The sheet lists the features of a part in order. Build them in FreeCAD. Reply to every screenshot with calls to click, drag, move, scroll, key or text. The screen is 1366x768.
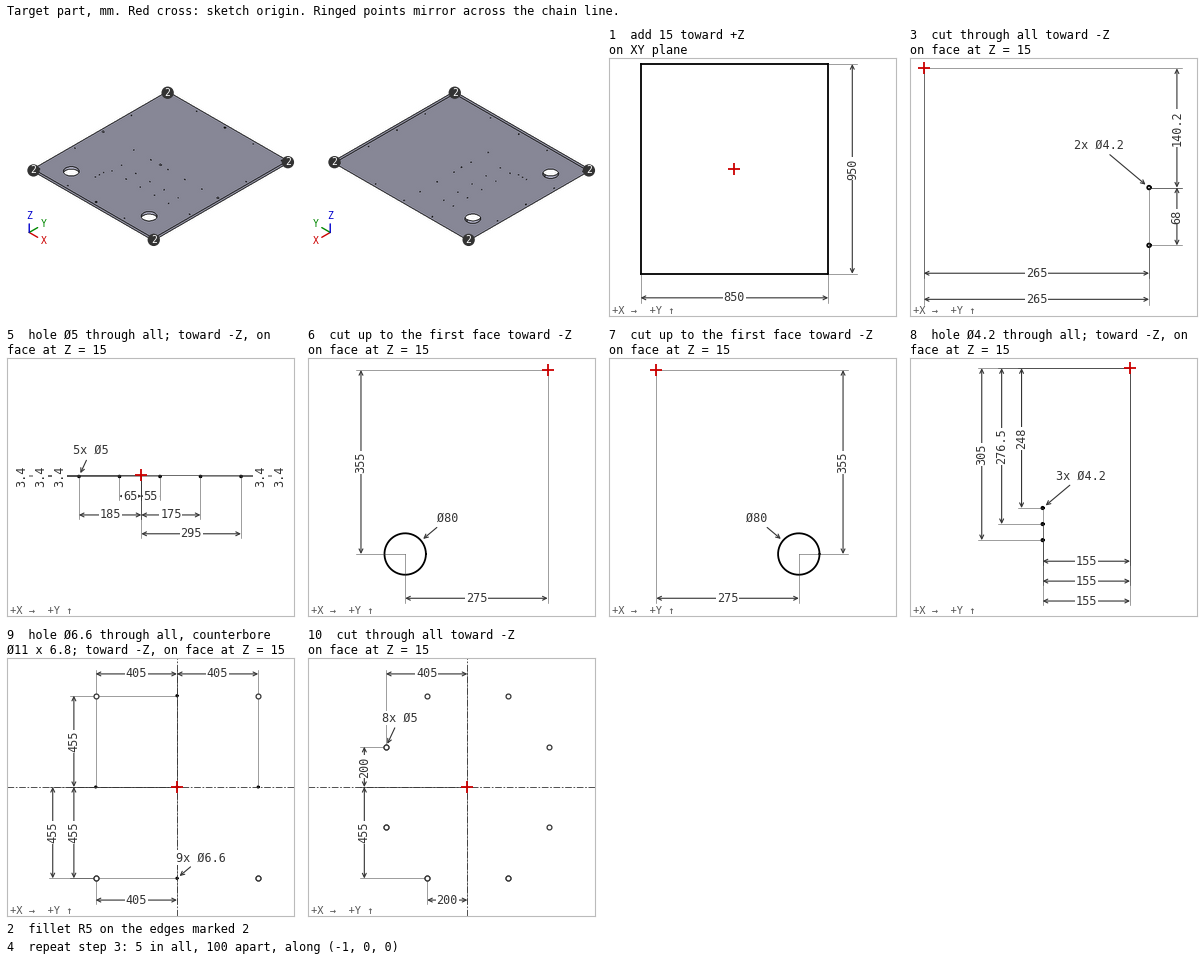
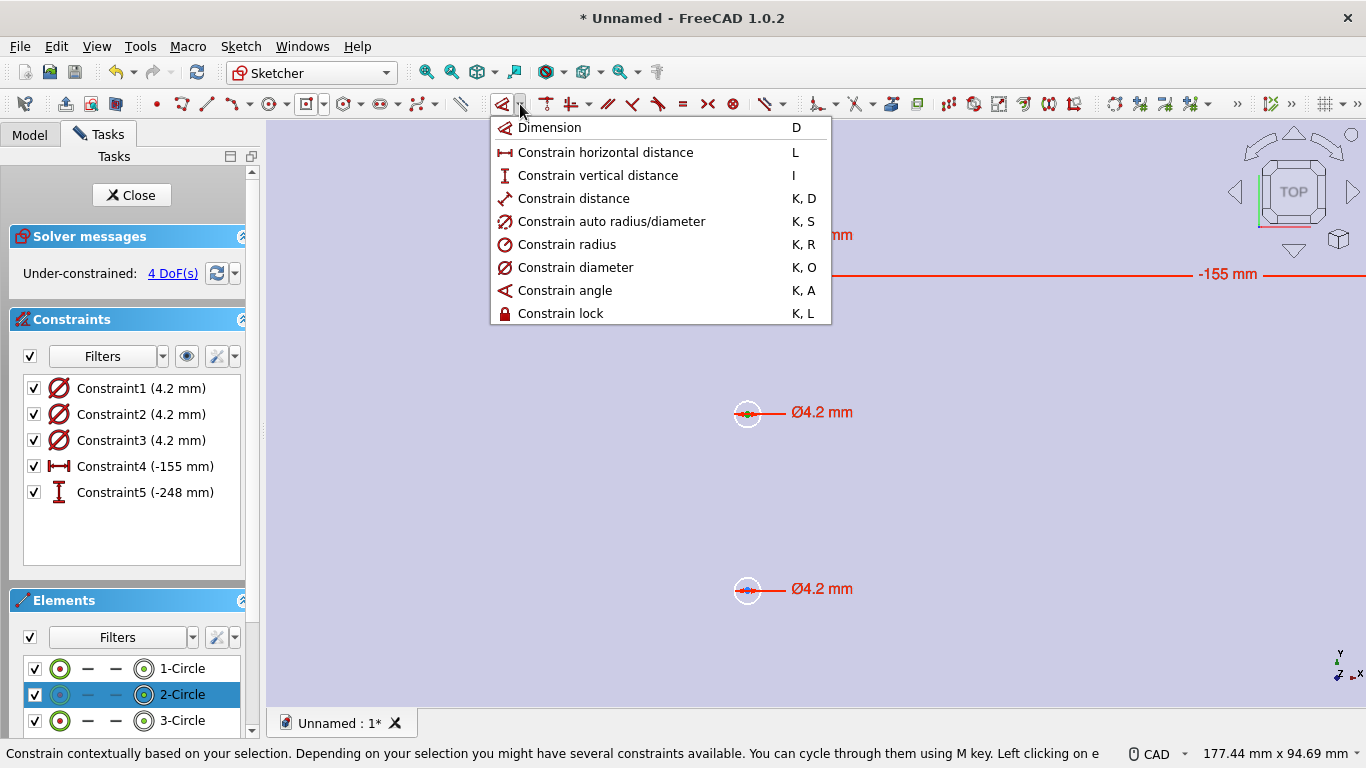
click(661, 152)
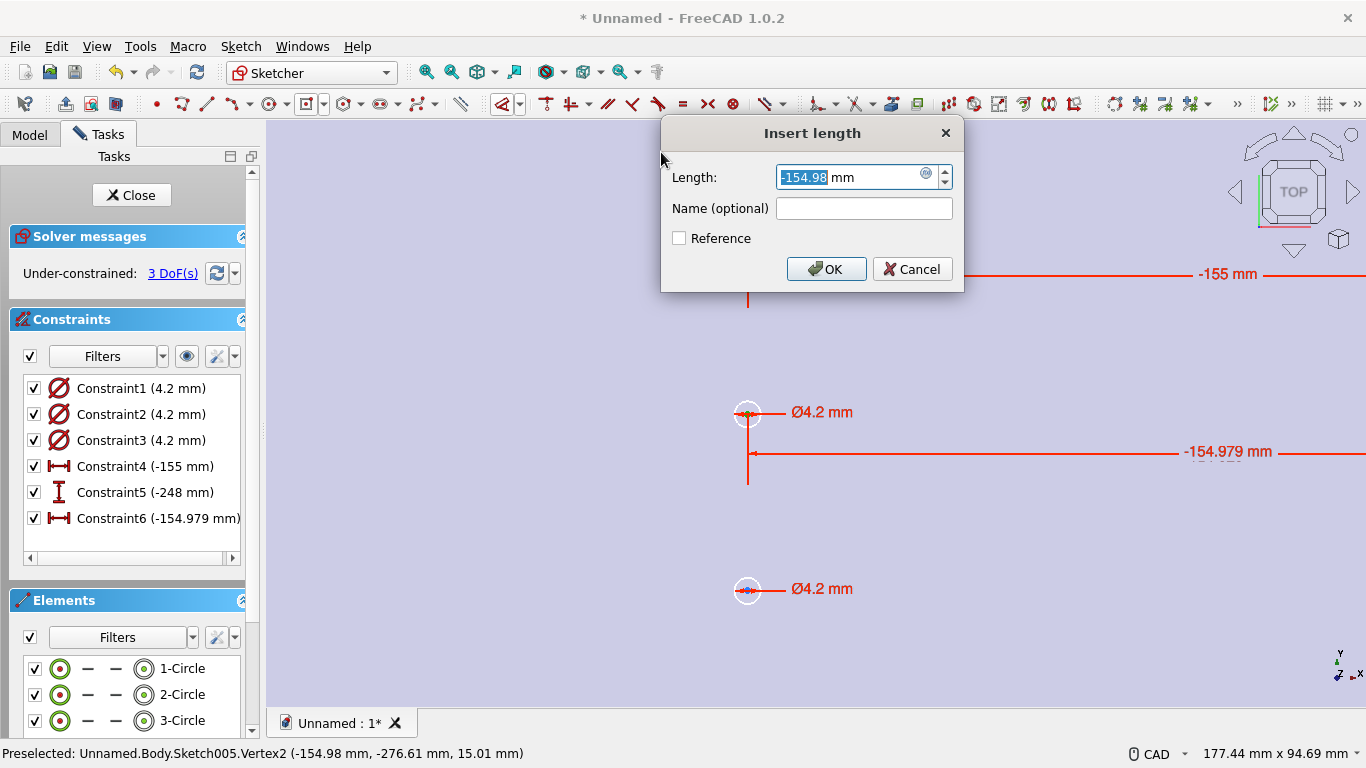
text(-155)
key(Return)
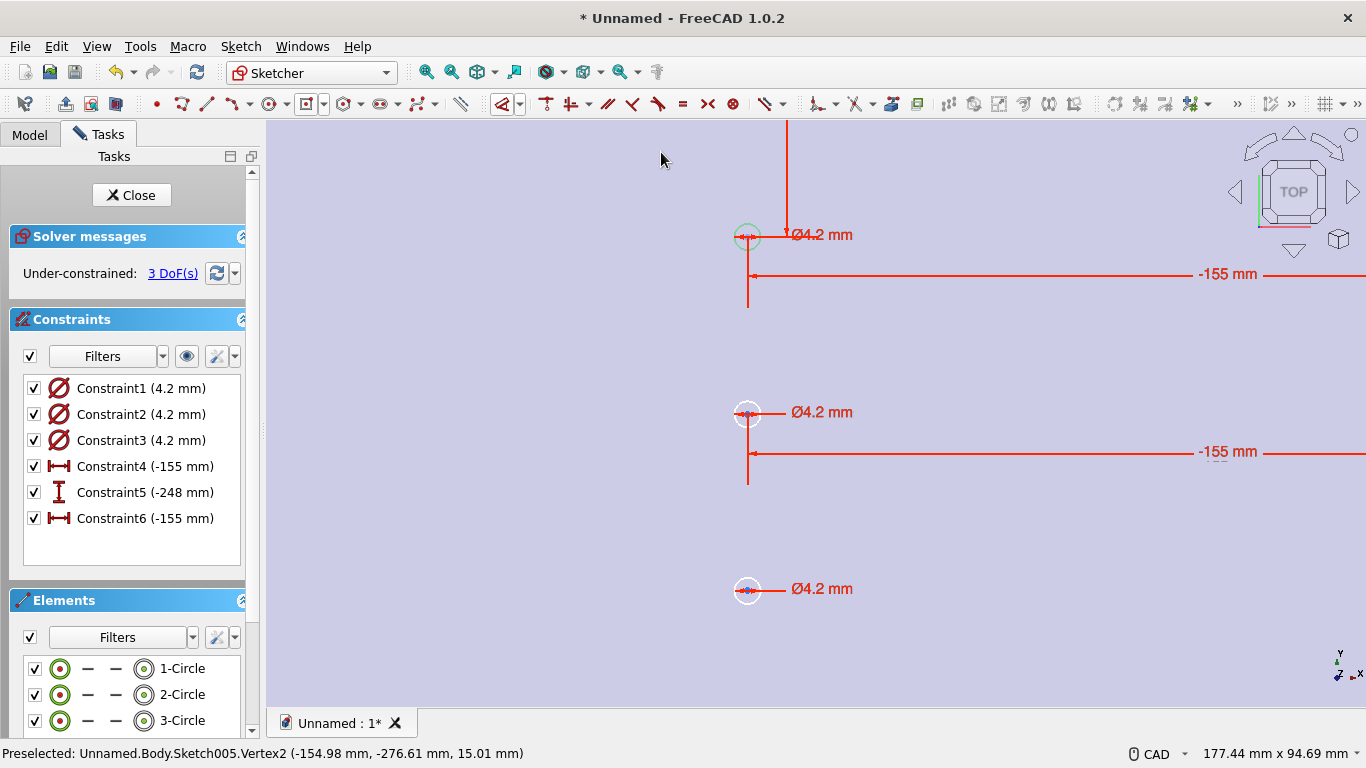
click(748, 591)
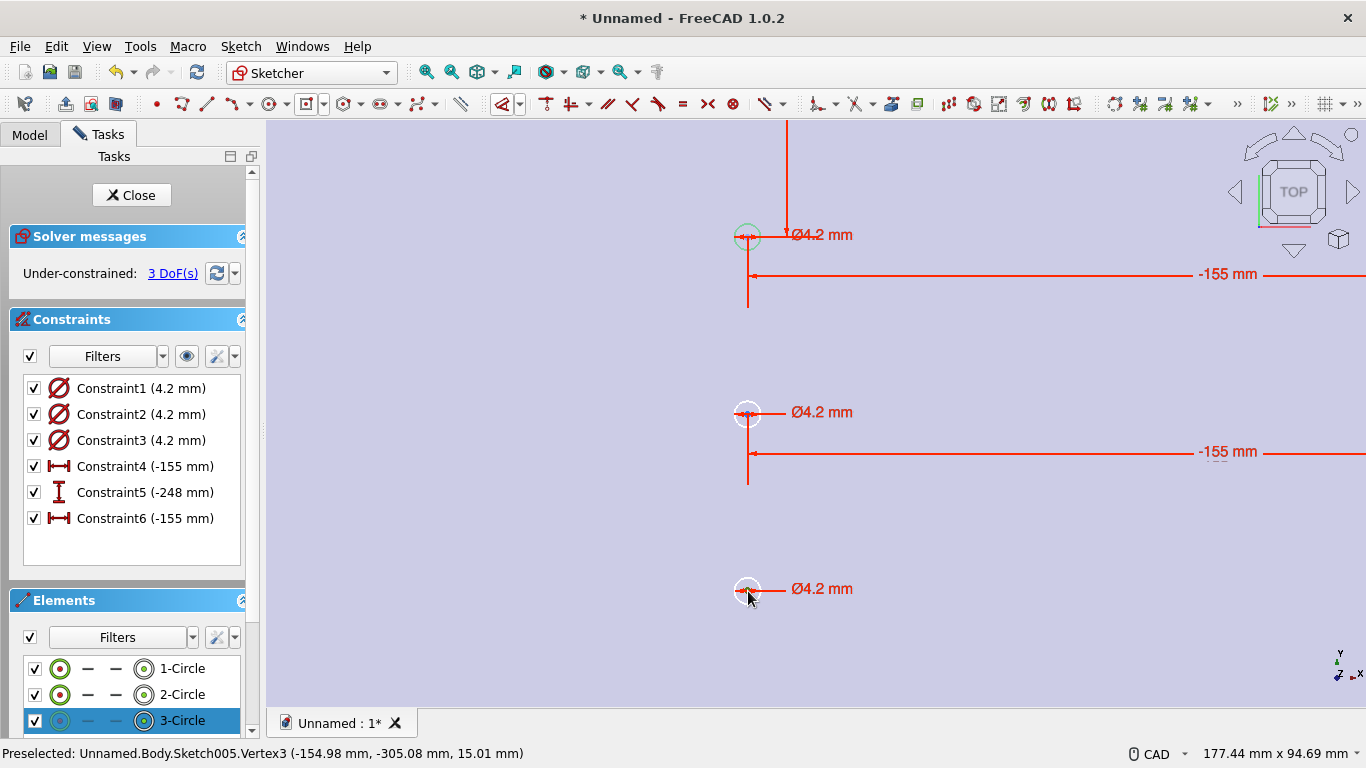
click(520, 104)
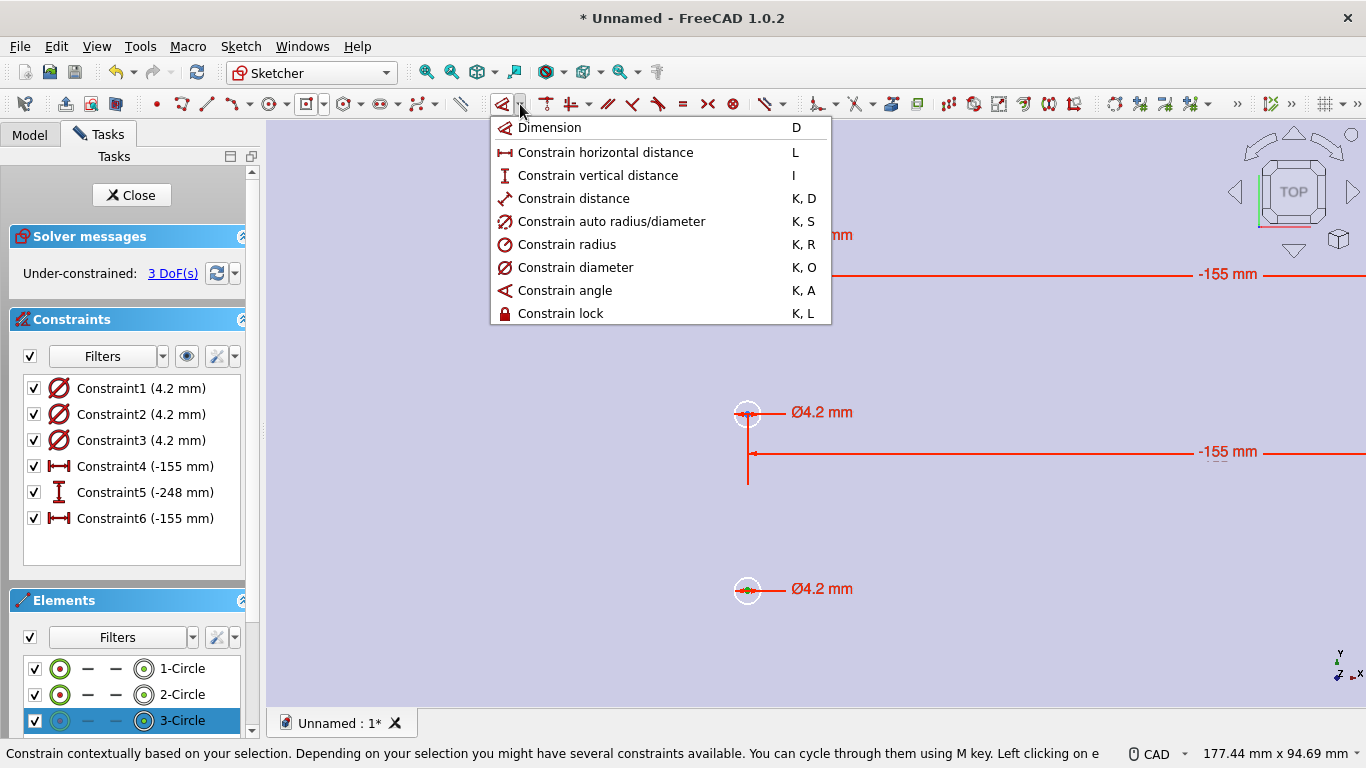
click(661, 152)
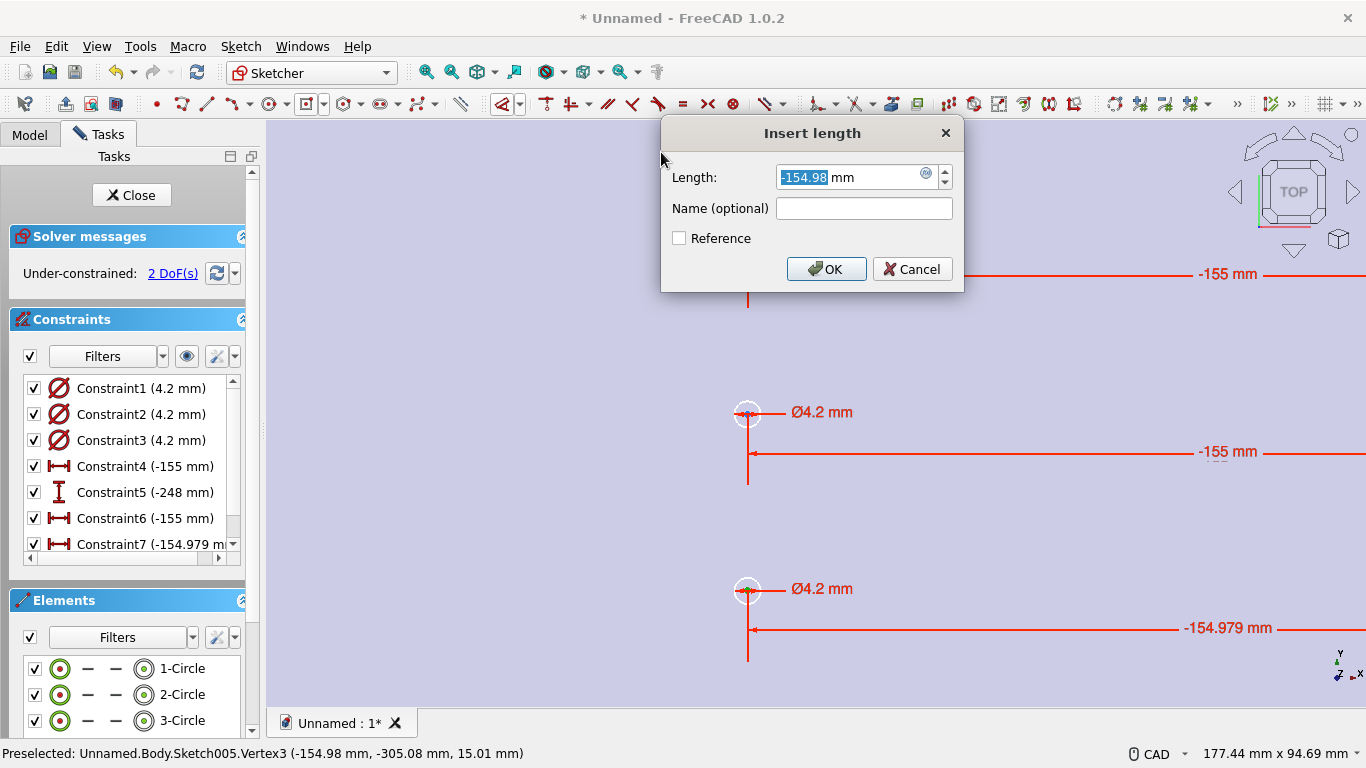
text(-155)
key(Return)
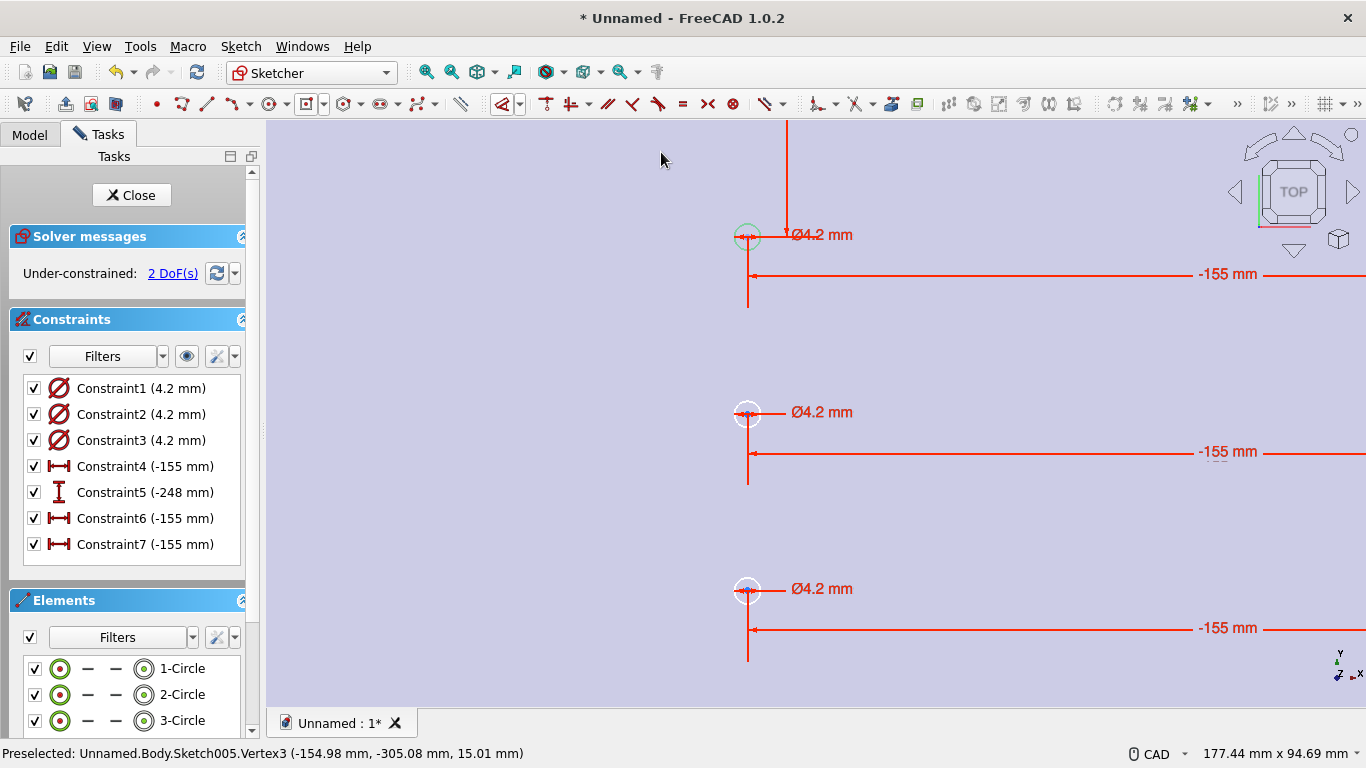
click(748, 591)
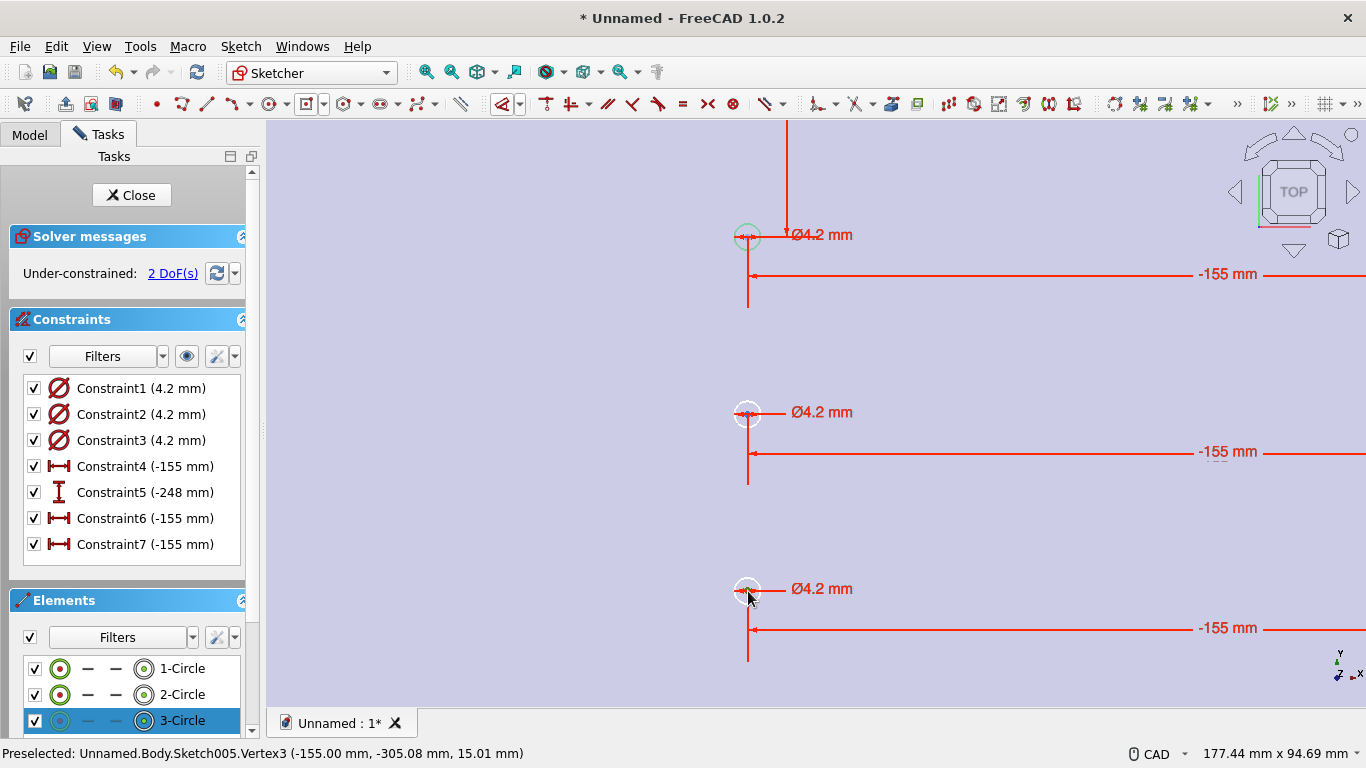
key(i)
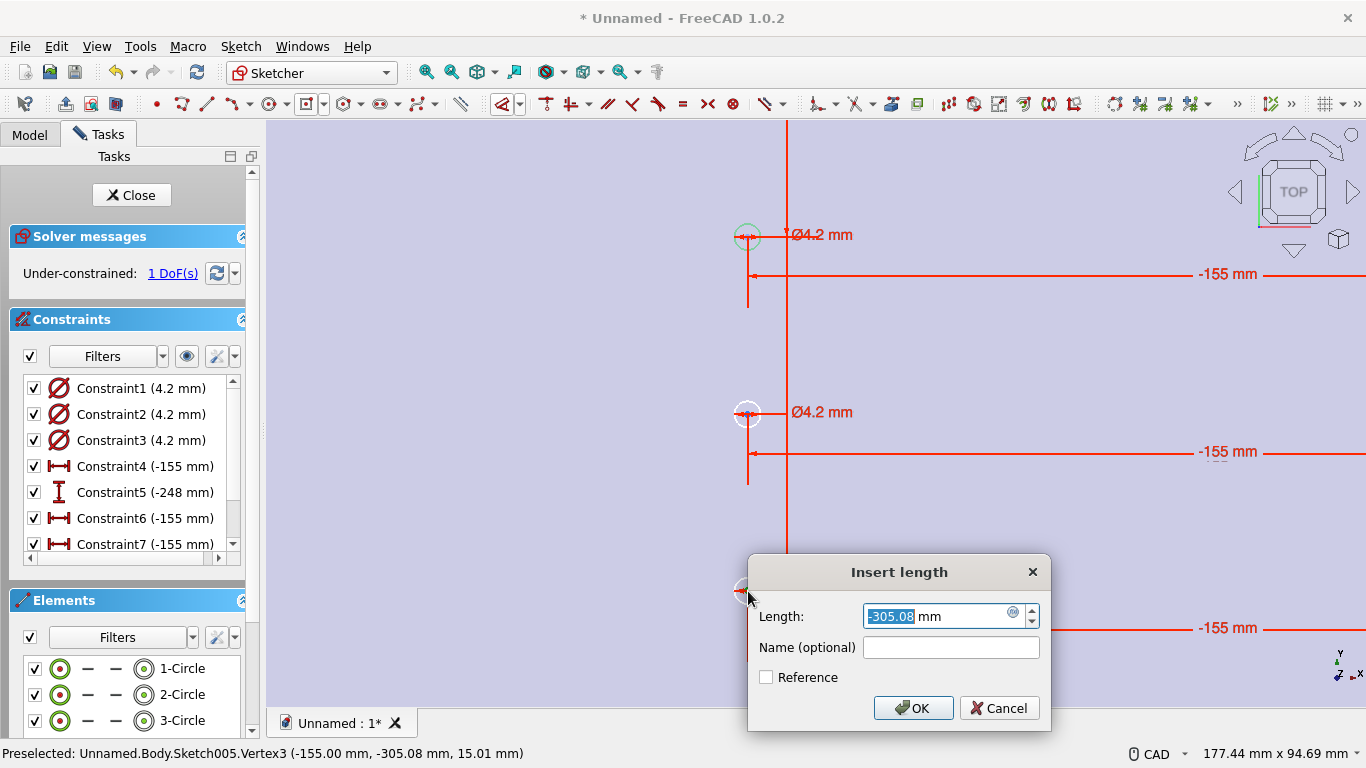
text(-305)
key(Return)